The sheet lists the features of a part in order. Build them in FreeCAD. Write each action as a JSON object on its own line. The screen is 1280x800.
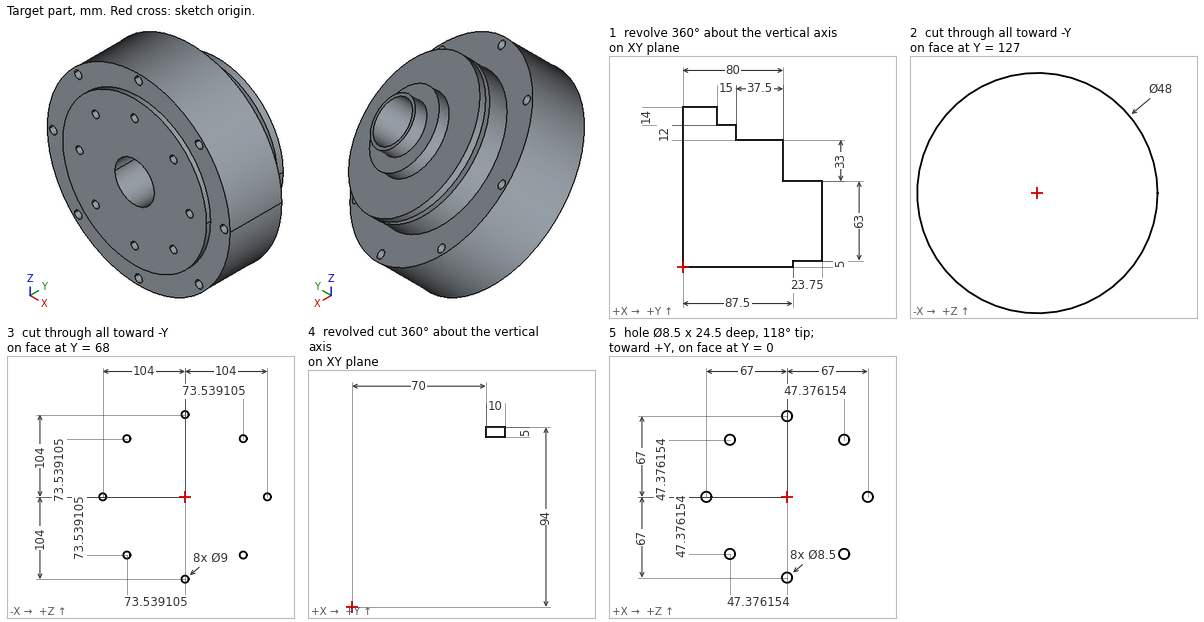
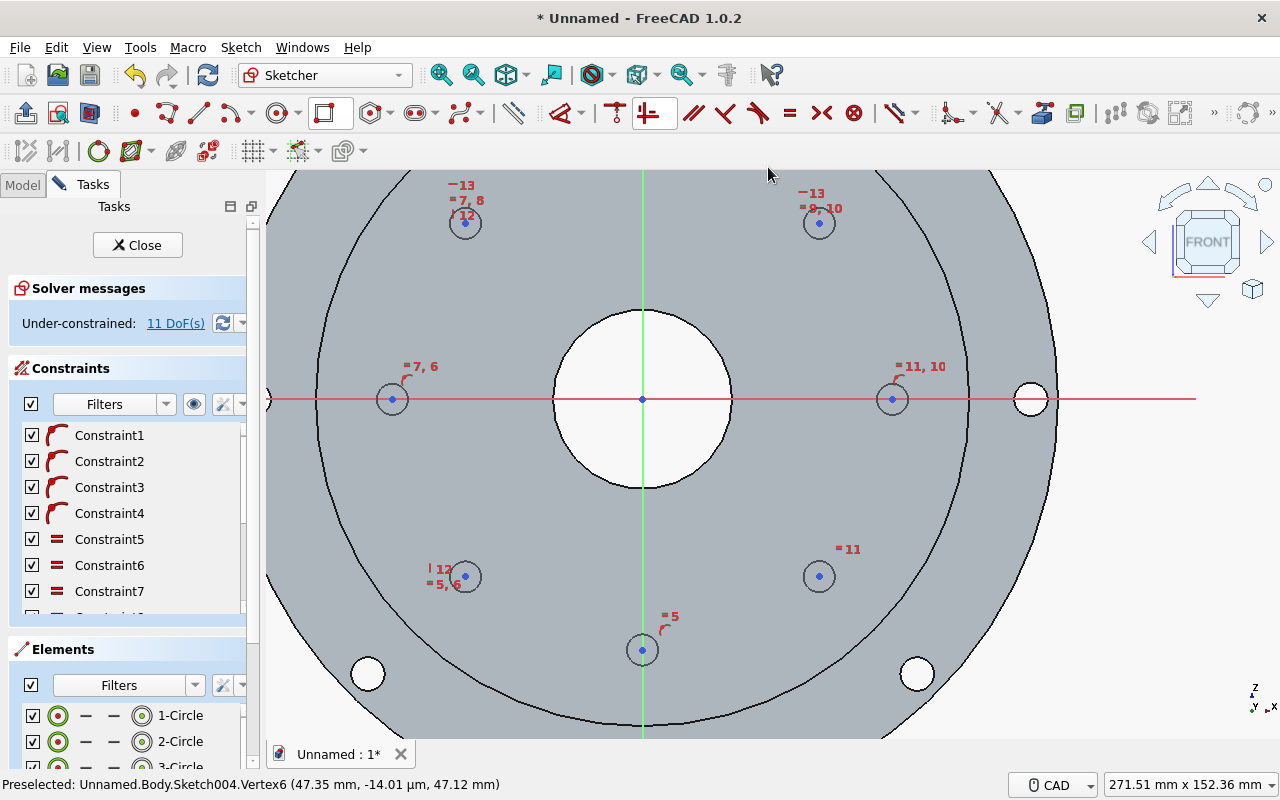
{"action": "left_click", "coordinate": [819, 223]}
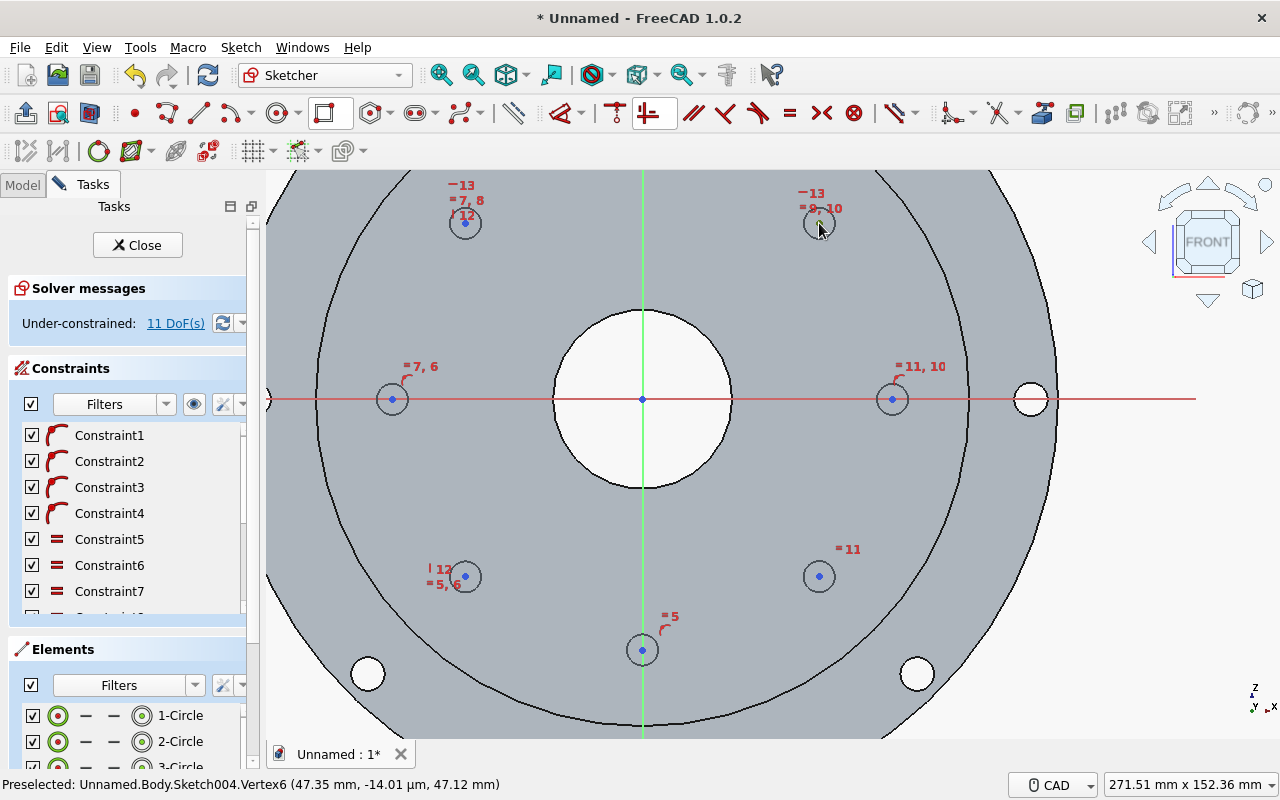
{"action": "left_click", "coordinate": [819, 577]}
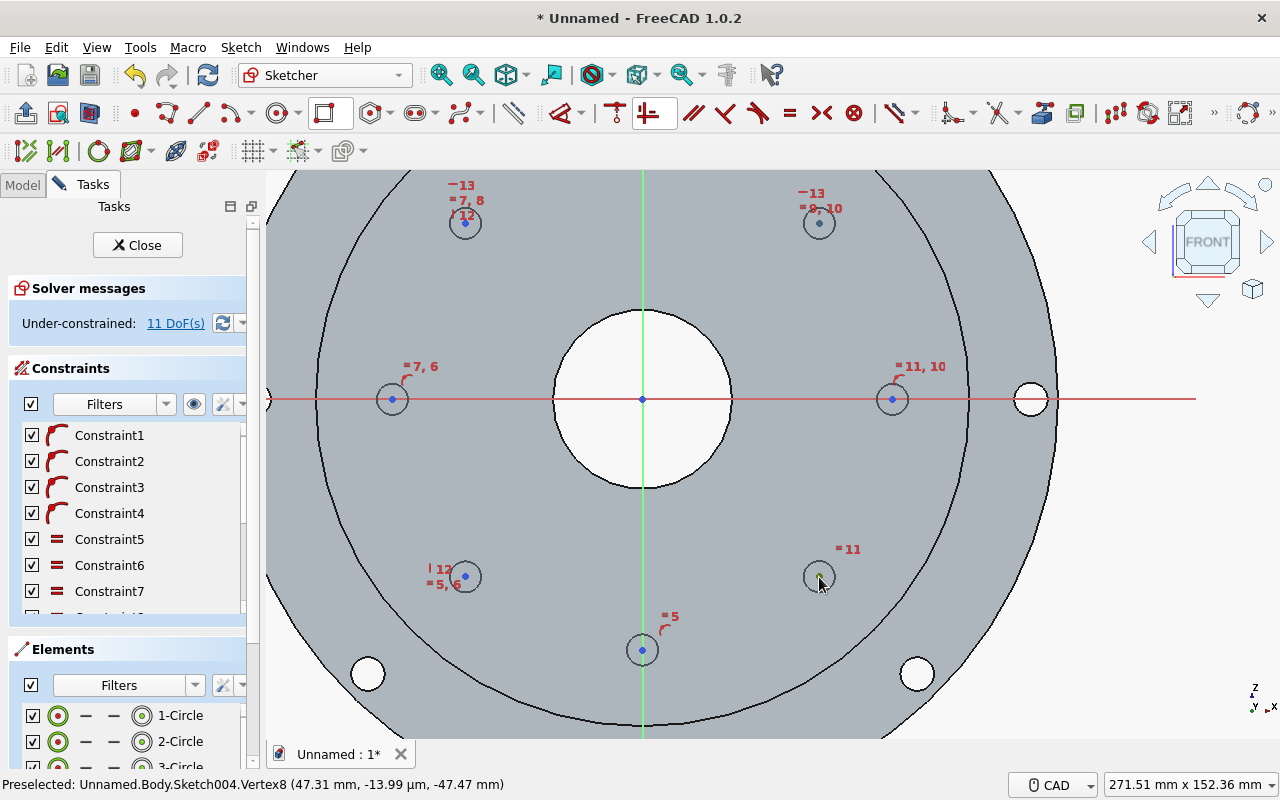
{"action": "left_click", "coordinate": [672, 114]}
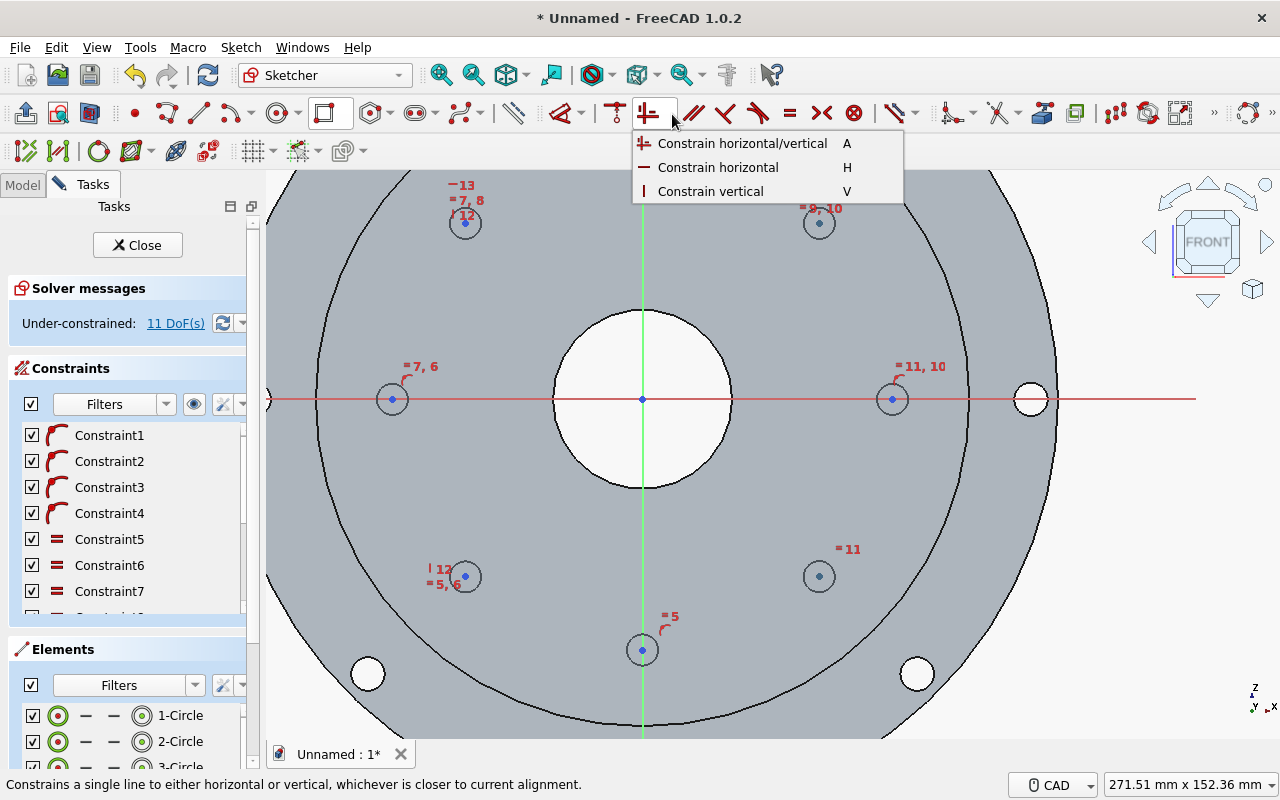
{"action": "left_click", "coordinate": [768, 191]}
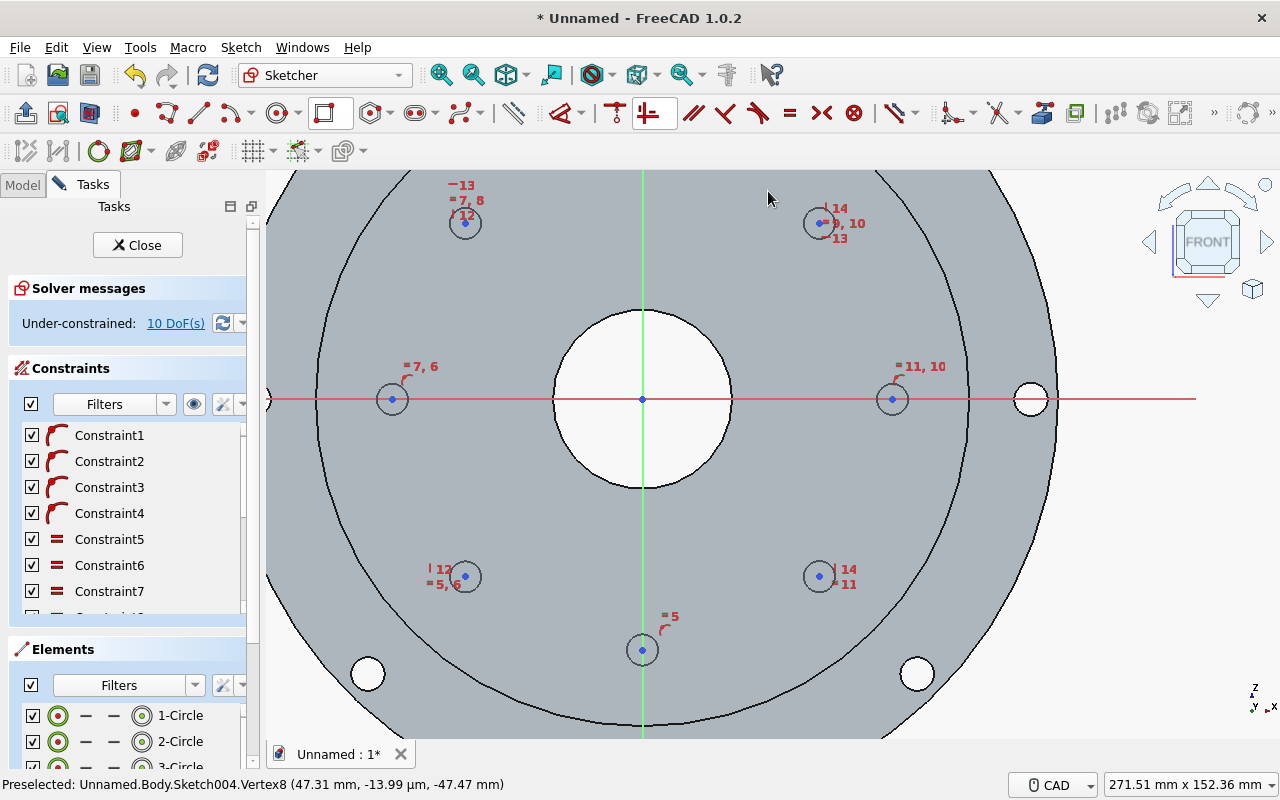
{"action": "left_click", "coordinate": [465, 577]}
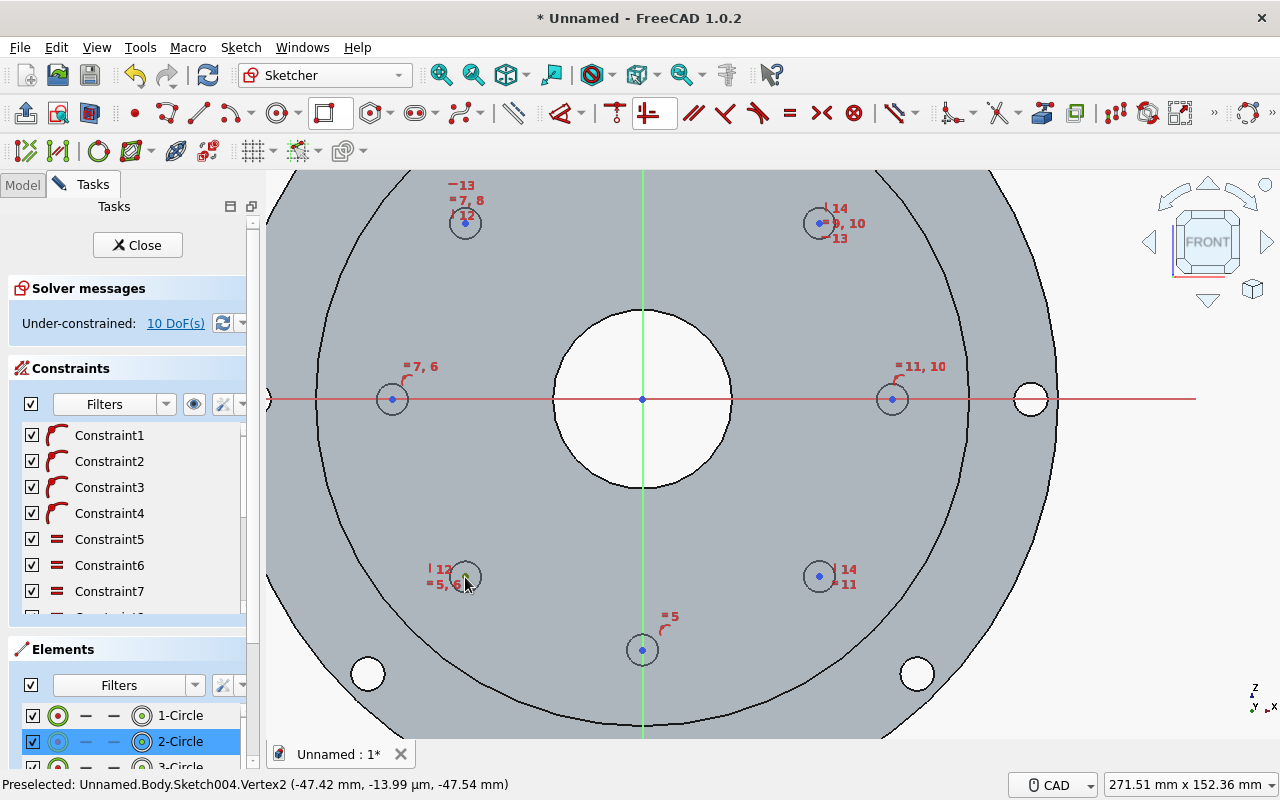
{"action": "left_click", "coordinate": [819, 577]}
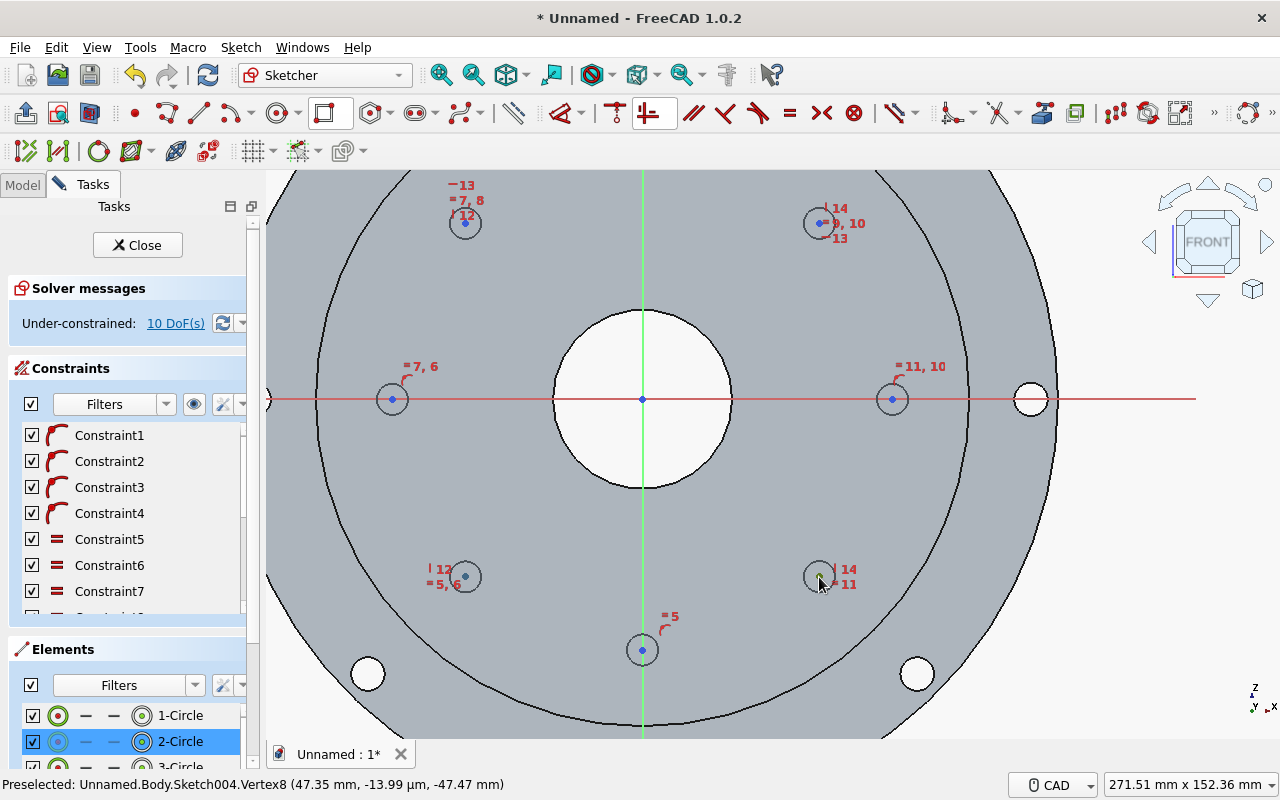
{"action": "key", "text": "h"}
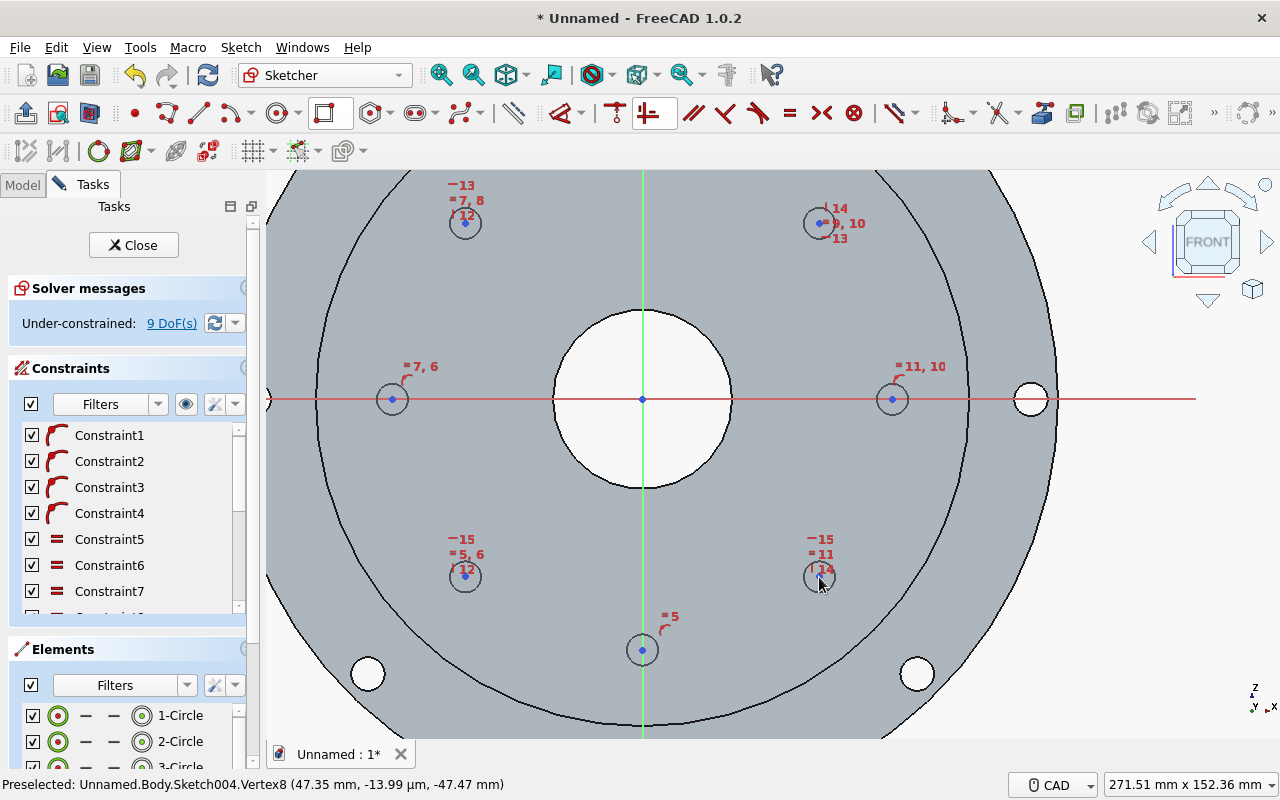
{"action": "left_click", "coordinate": [560, 114]}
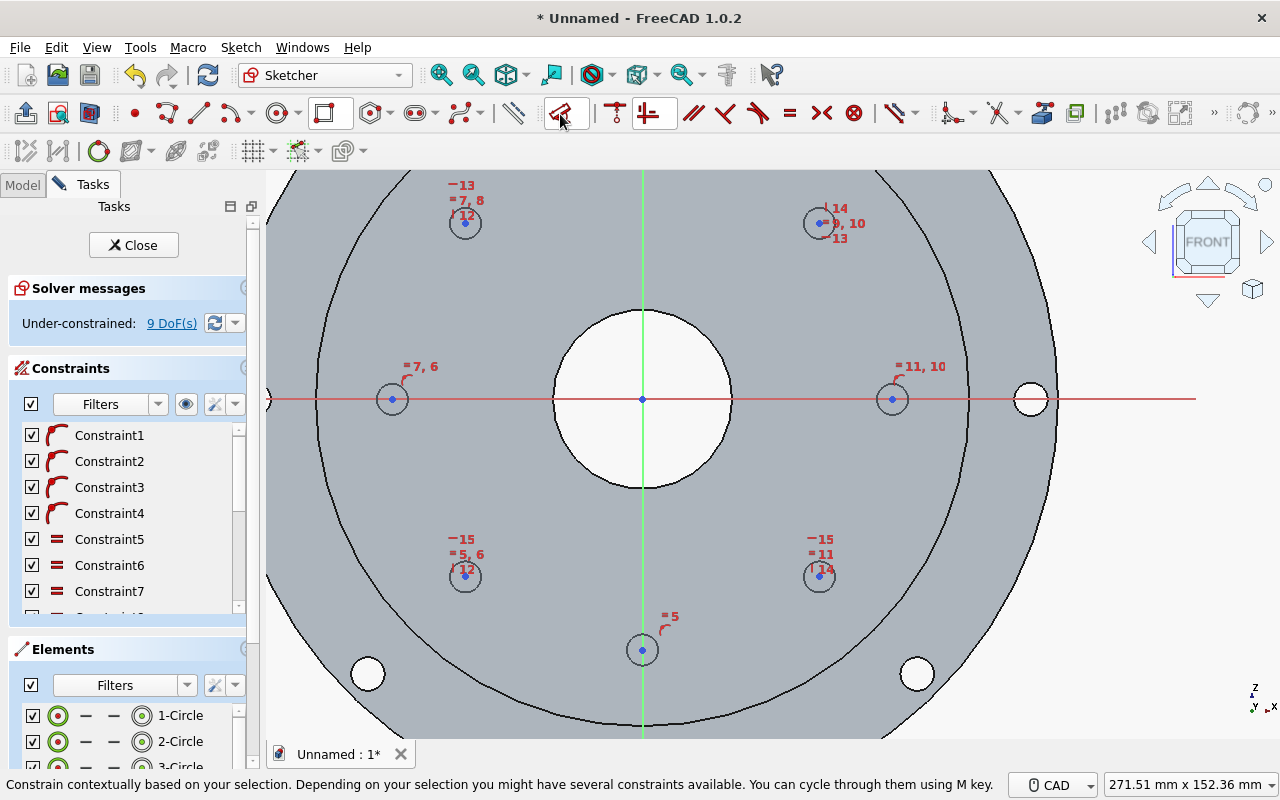
{"action": "scroll", "coordinate": [654, 639], "scroll_direction": "up", "scroll_amount": 2}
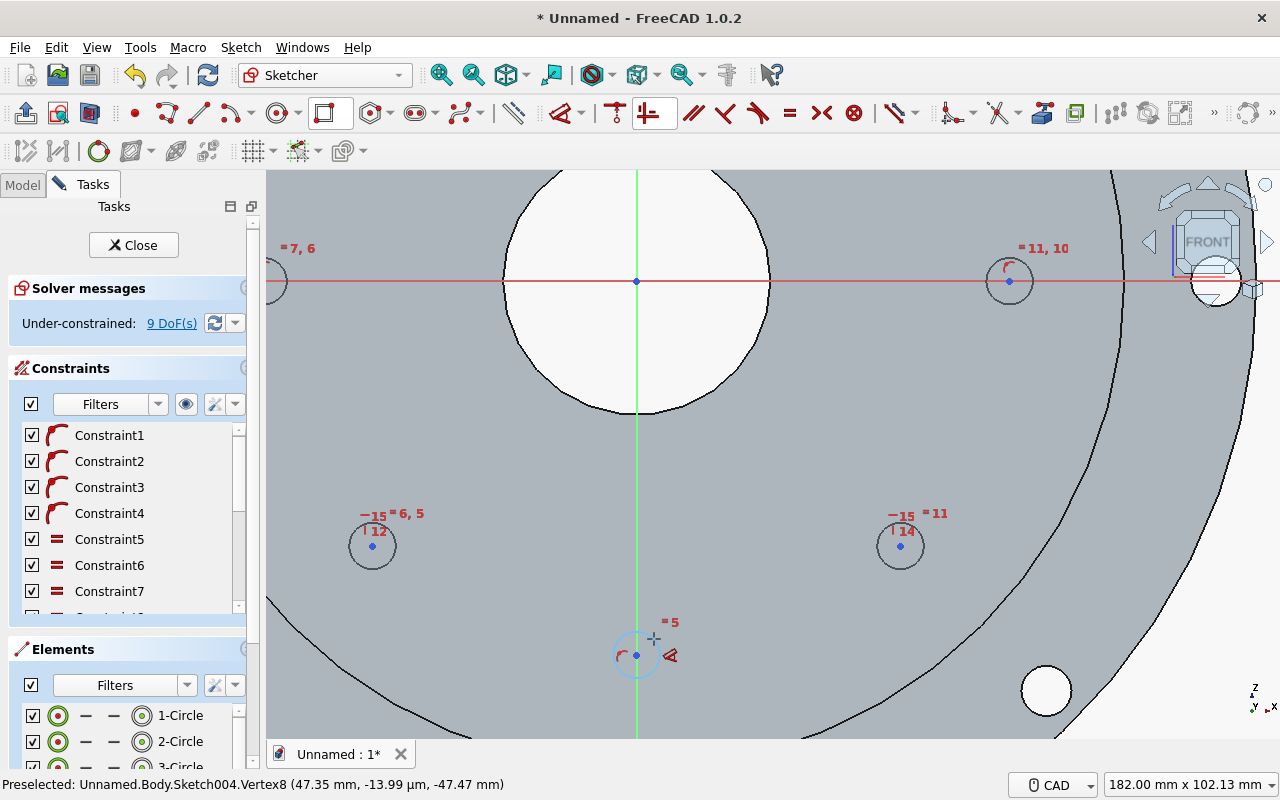
{"action": "left_click", "coordinate": [653, 639]}
{"action": "left_click", "coordinate": [676, 617]}